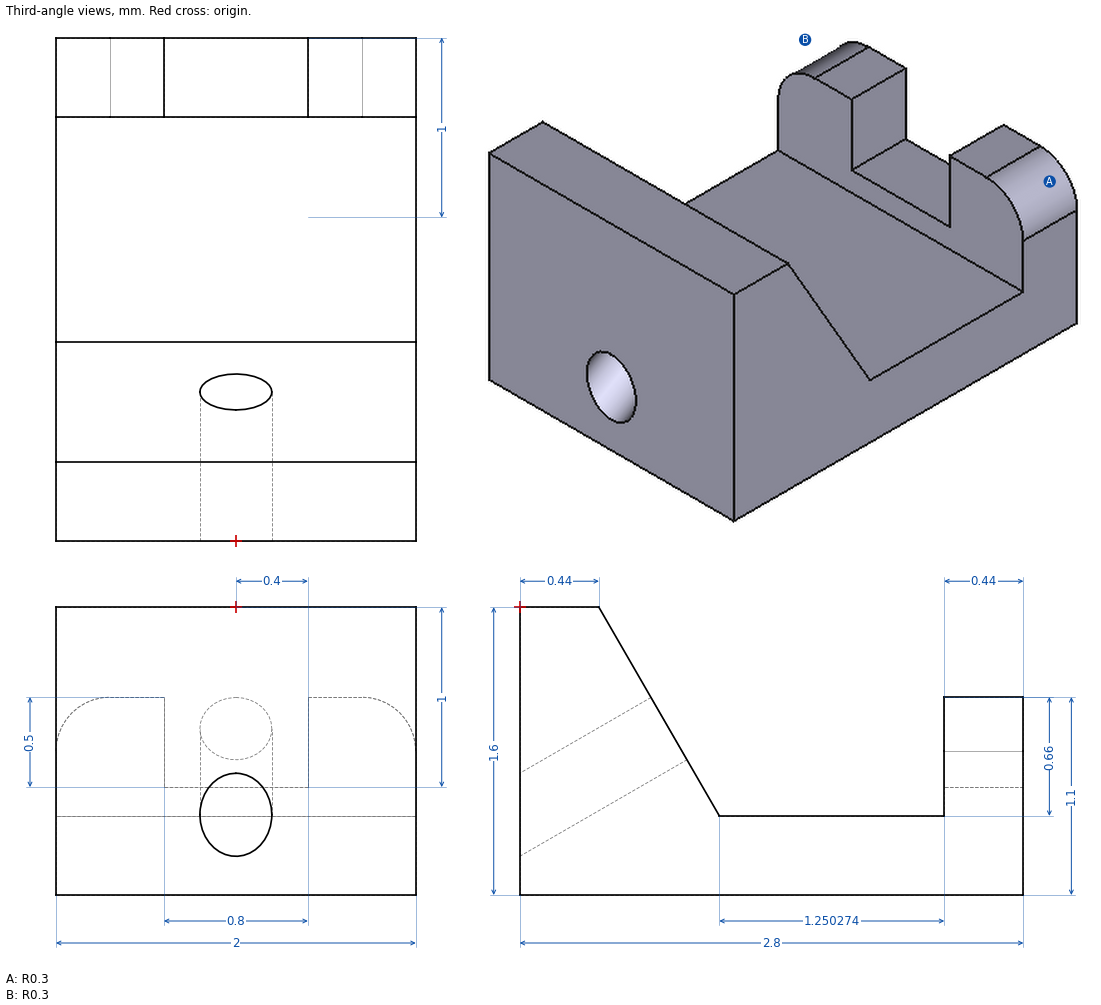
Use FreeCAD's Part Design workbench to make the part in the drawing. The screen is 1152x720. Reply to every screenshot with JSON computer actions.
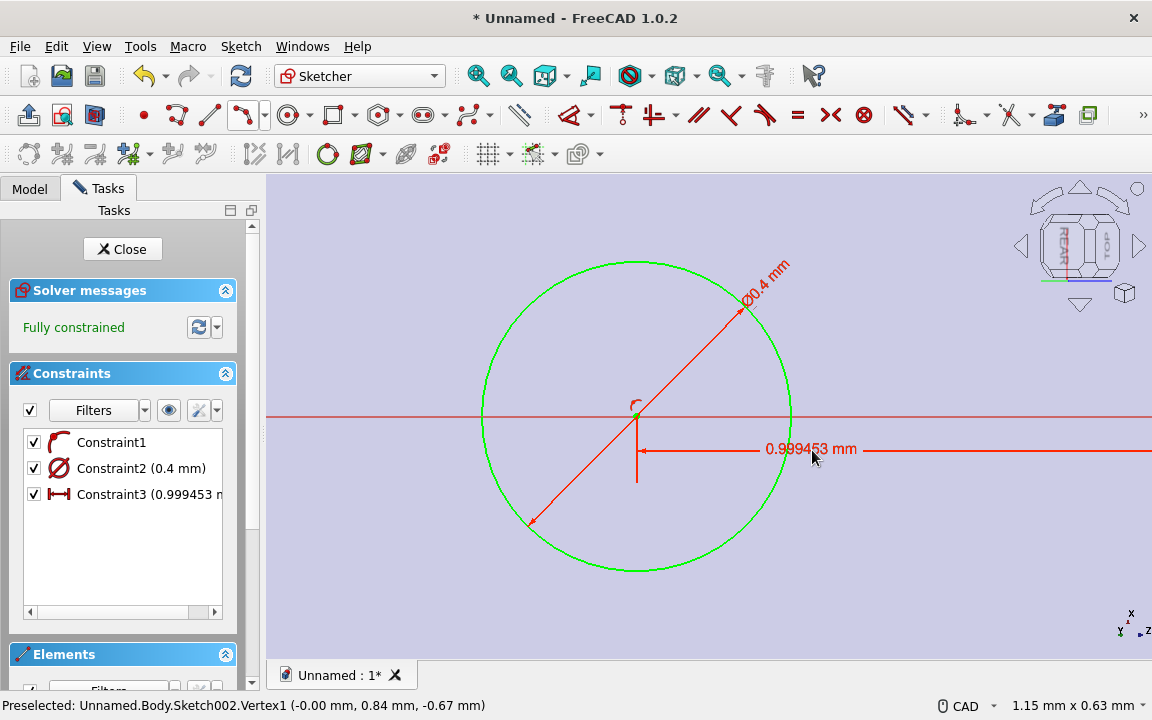
{"action": "left_click", "coordinate": [123, 249]}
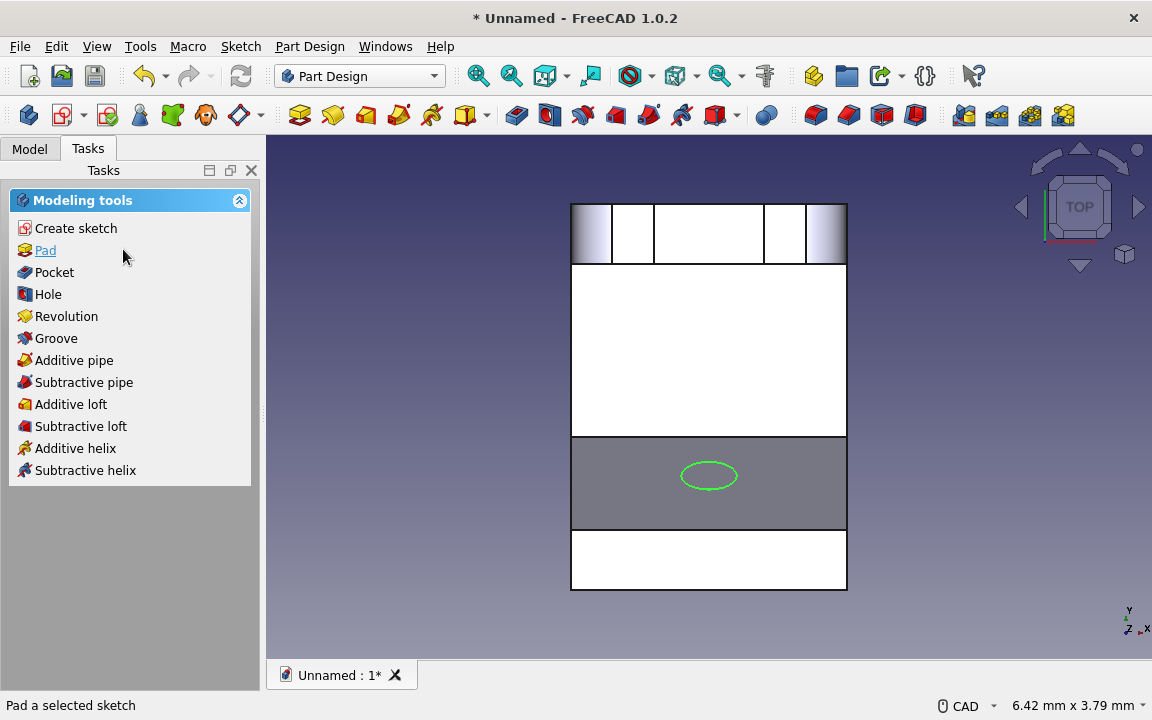
{"action": "left_click", "coordinate": [517, 116]}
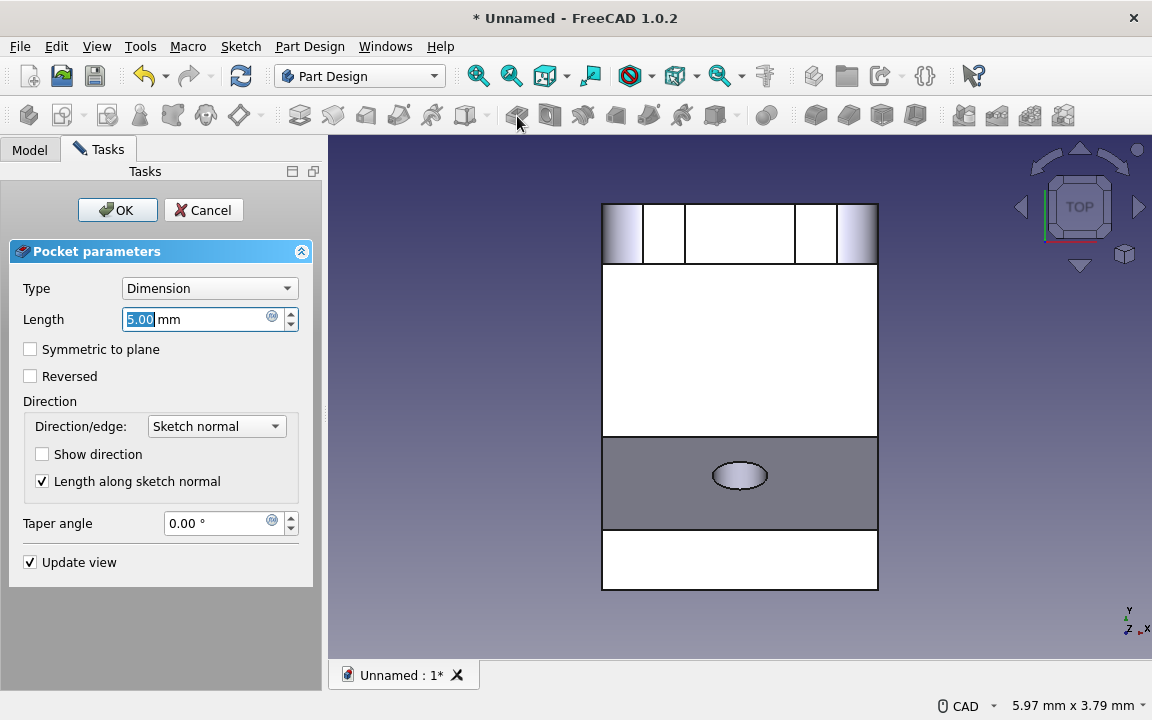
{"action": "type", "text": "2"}
{"action": "key", "text": "Tab"}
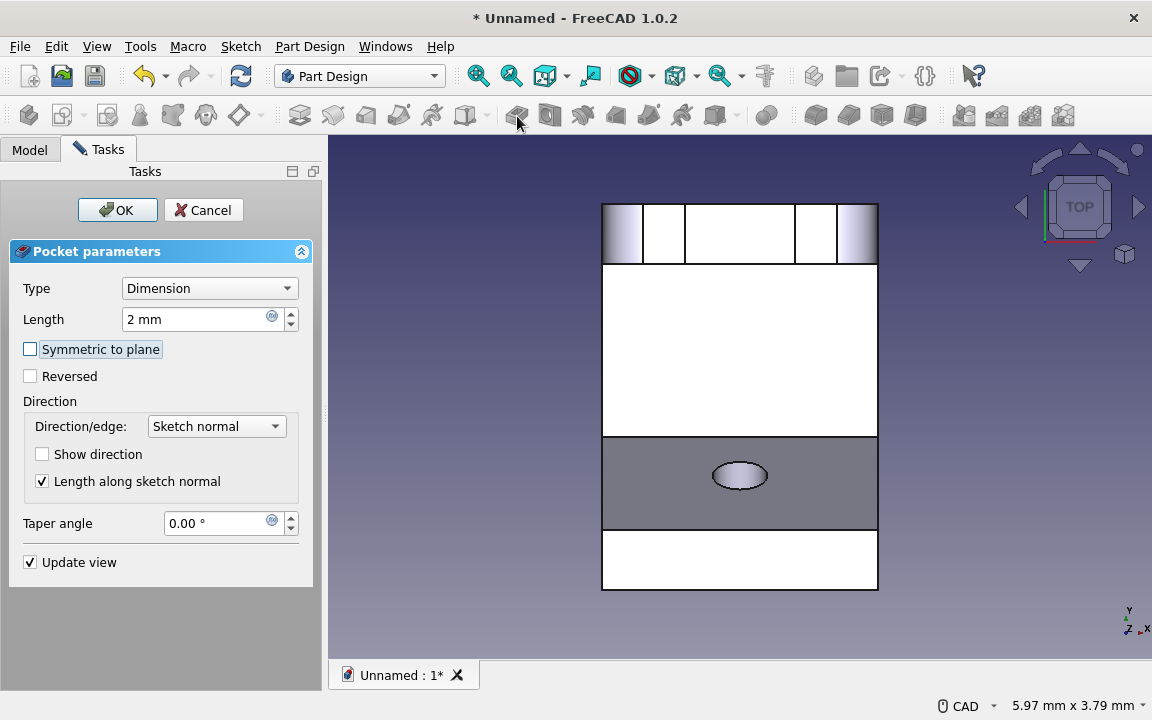
{"action": "left_click", "coordinate": [118, 210]}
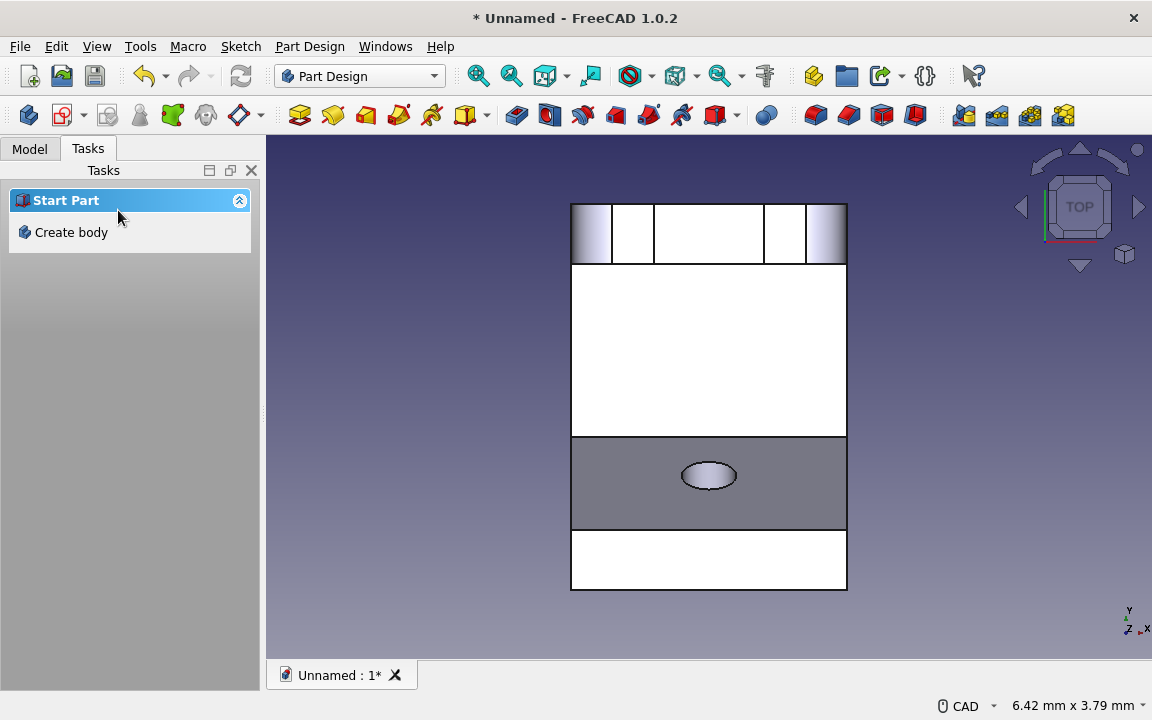
{"action": "key", "text": "0"}